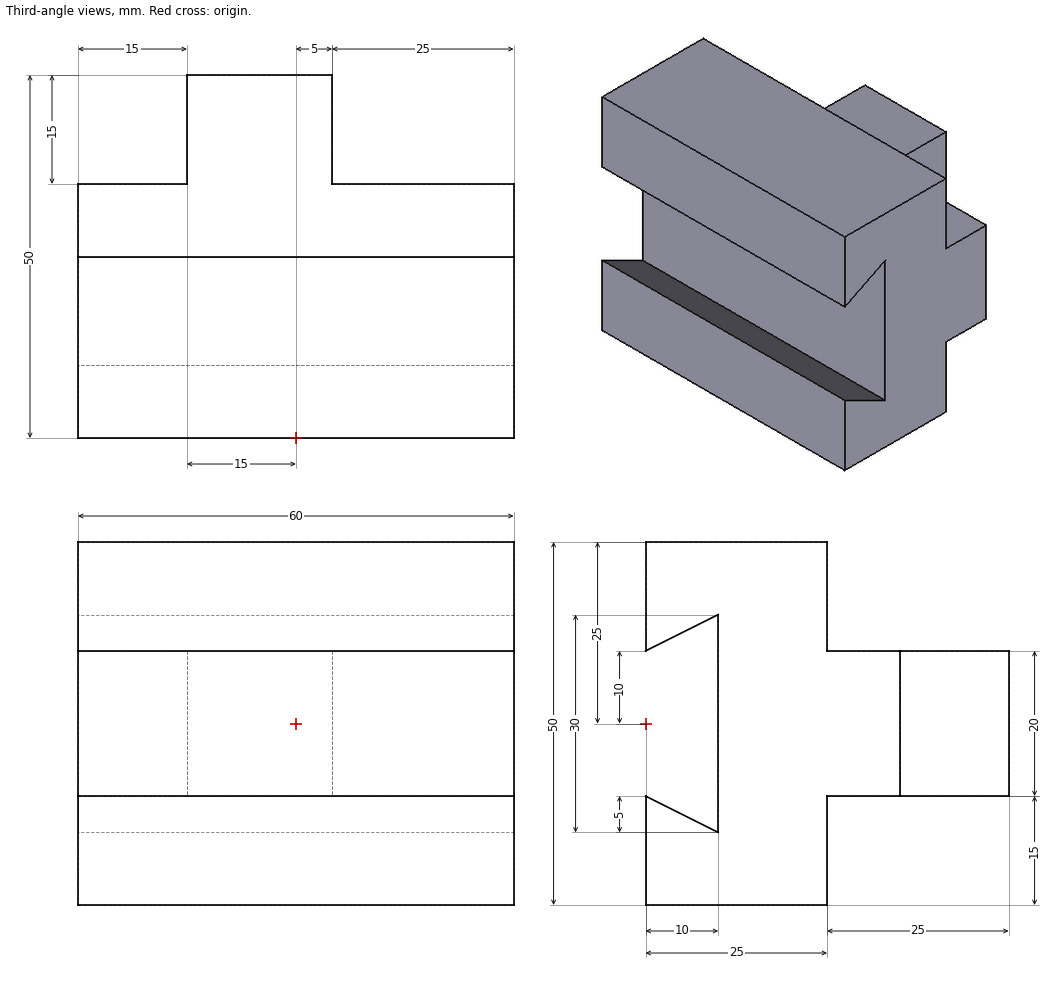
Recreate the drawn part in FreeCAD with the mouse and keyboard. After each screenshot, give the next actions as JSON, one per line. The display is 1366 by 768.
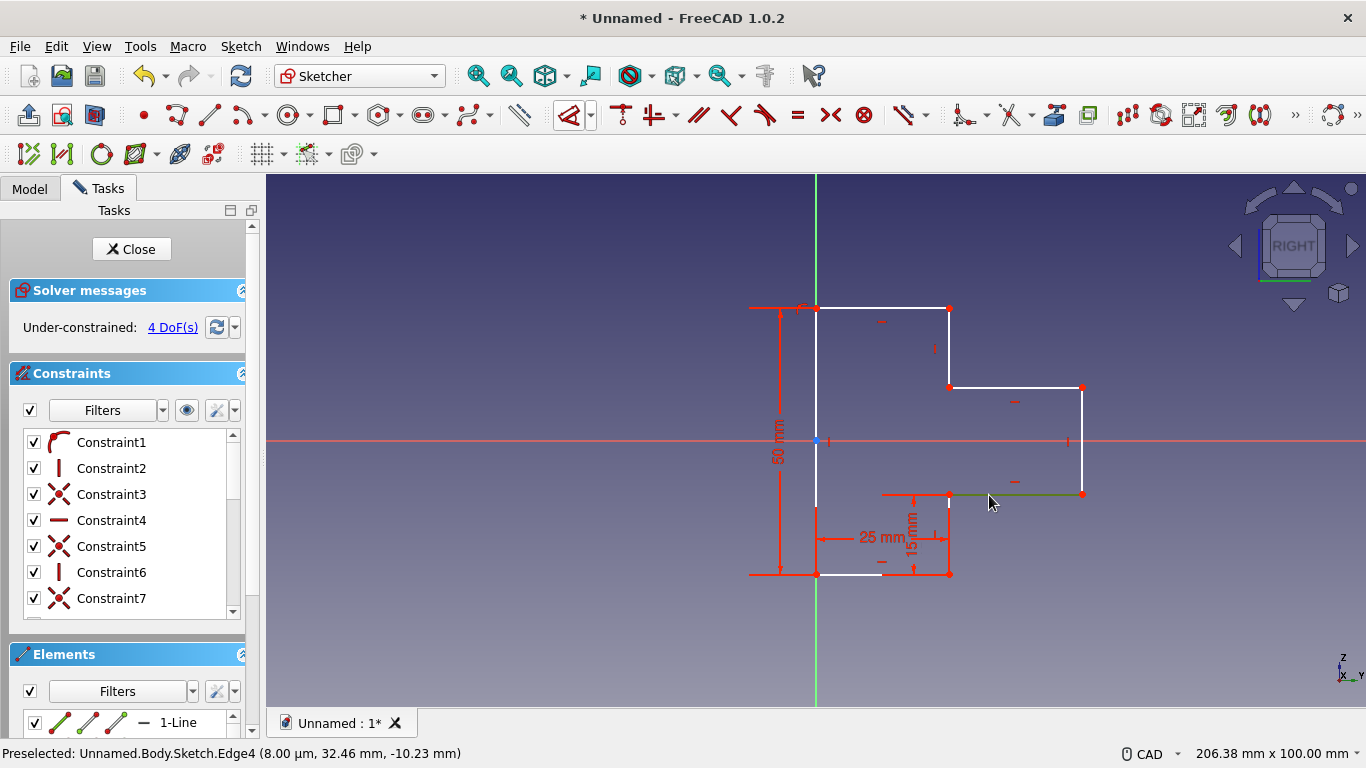
{"action": "key", "text": "l"}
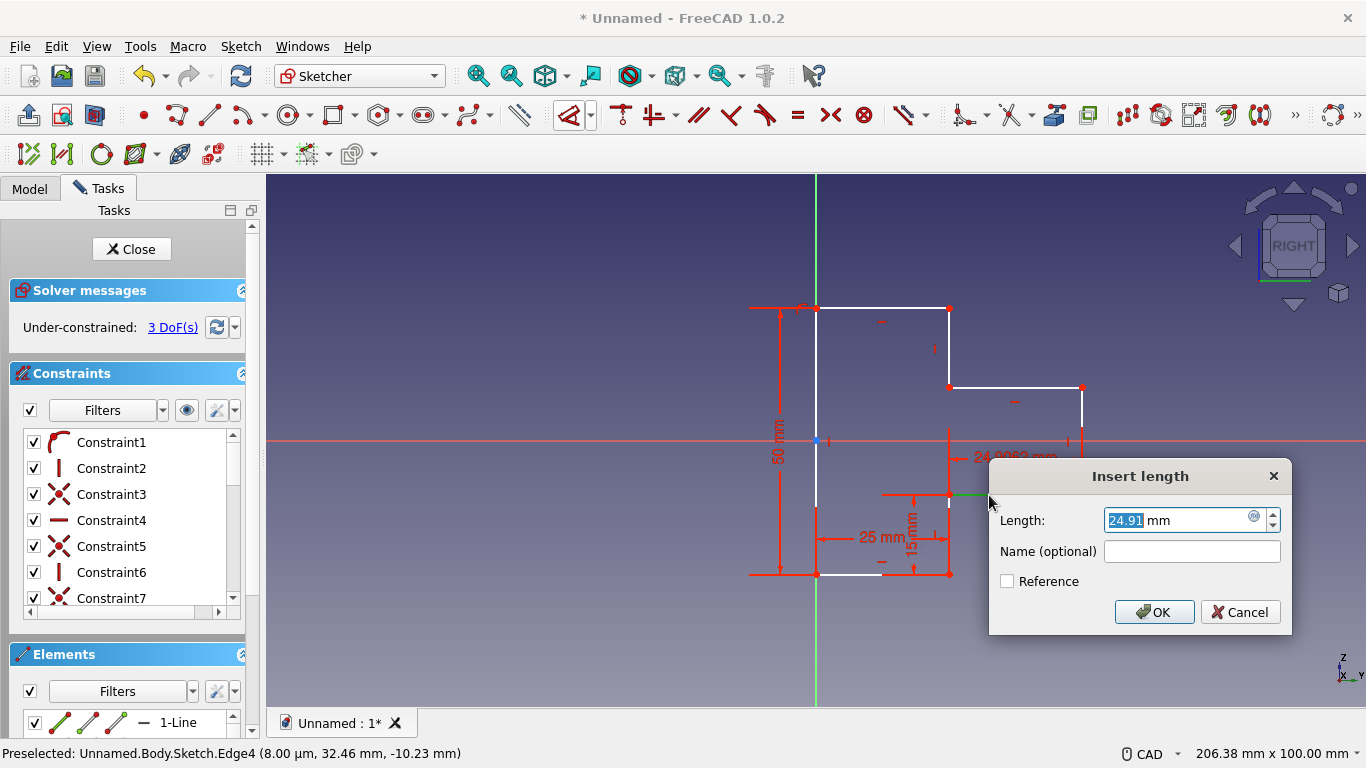
{"action": "type", "text": "25"}
{"action": "key", "text": "Return"}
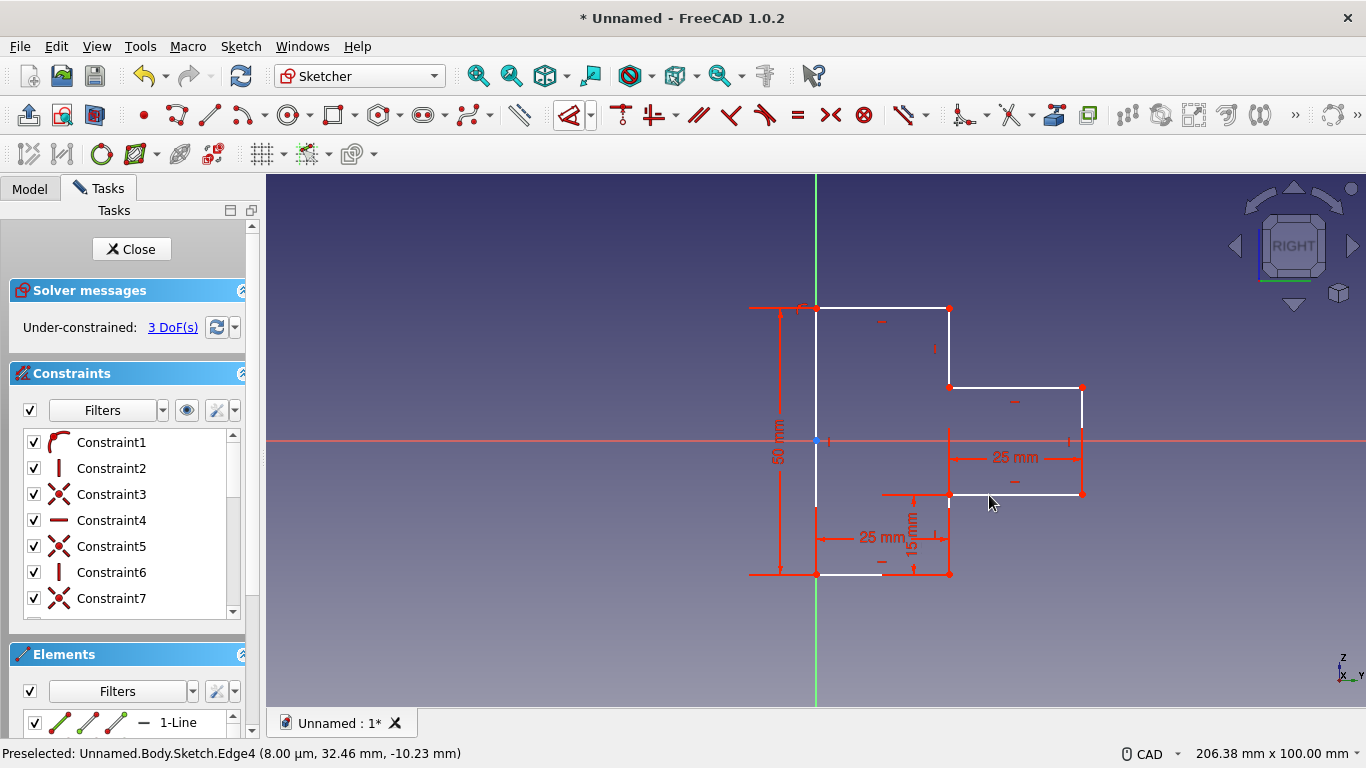
{"action": "left_click", "coordinate": [1082, 463]}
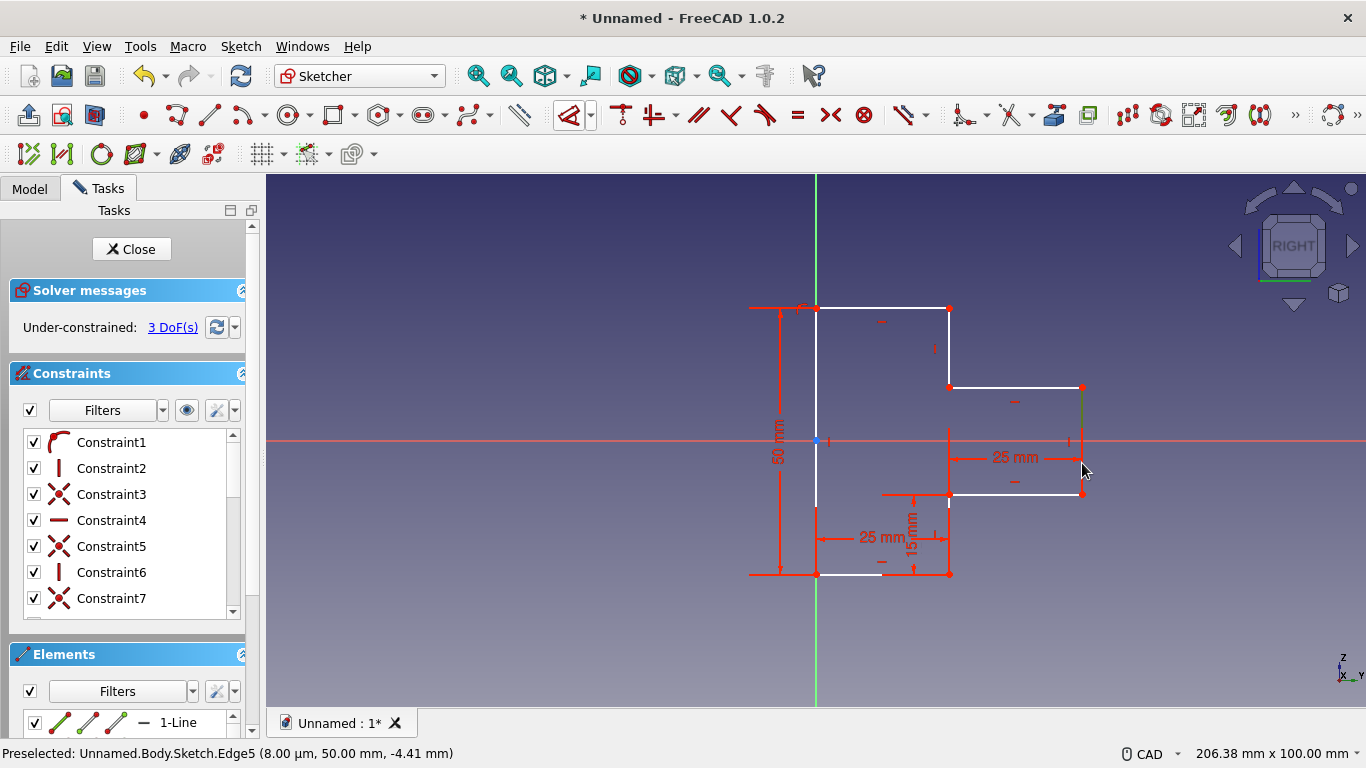
{"action": "left_click", "coordinate": [590, 116]}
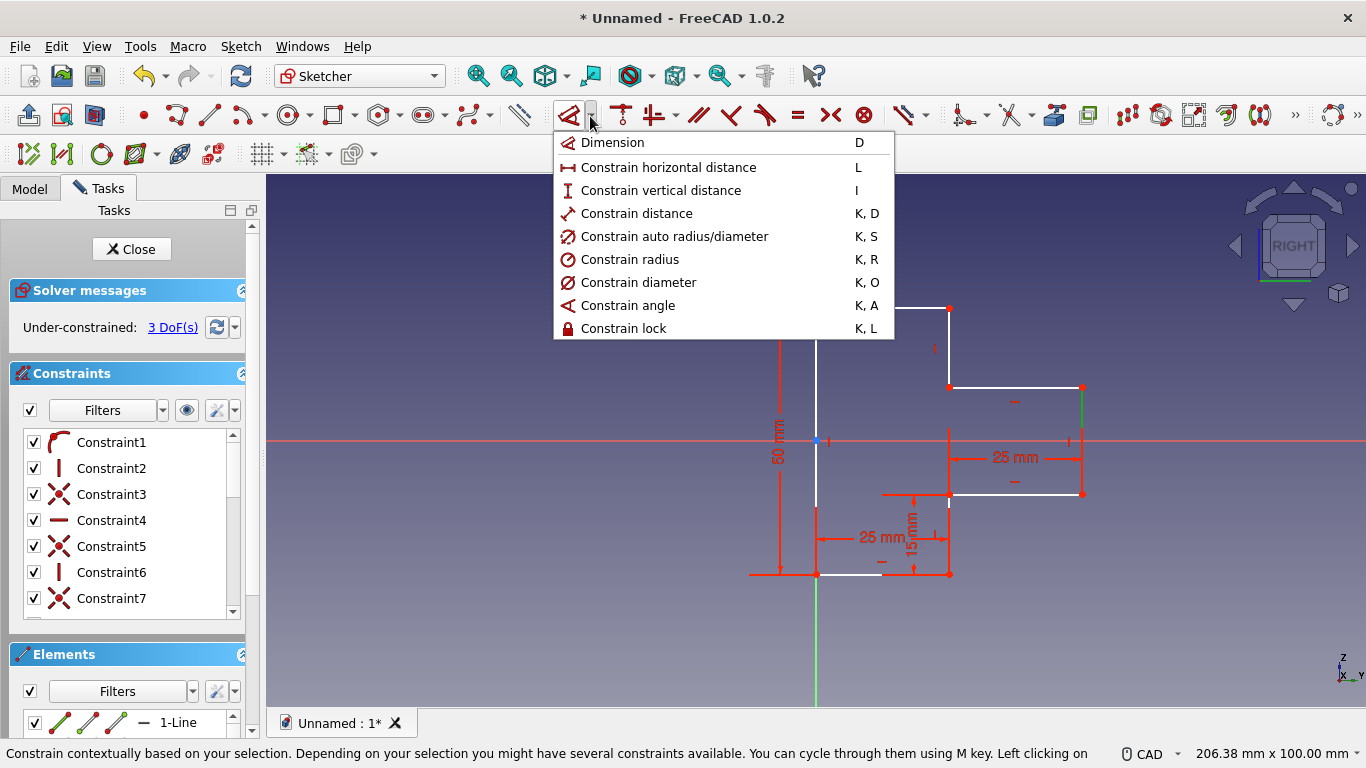
{"action": "left_click", "coordinate": [724, 190]}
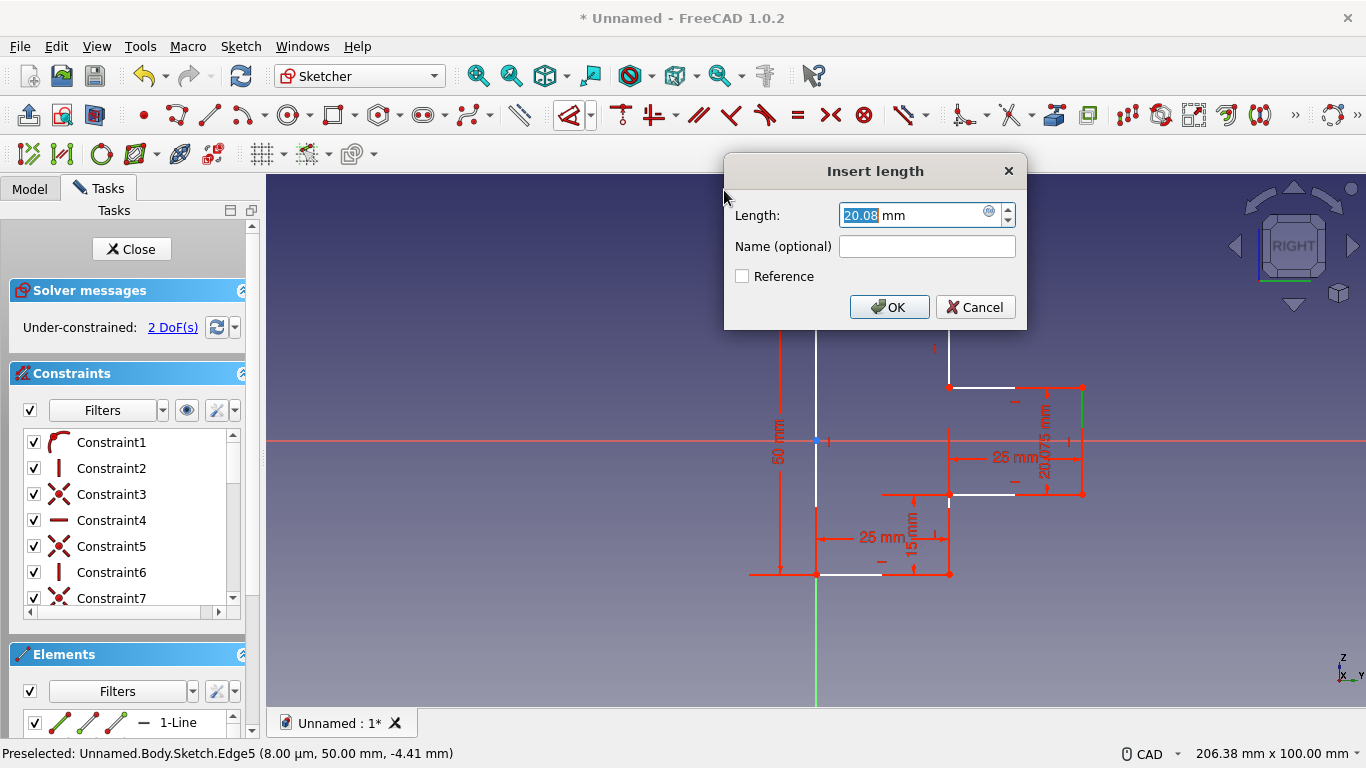
{"action": "type", "text": "20"}
{"action": "key", "text": "Return"}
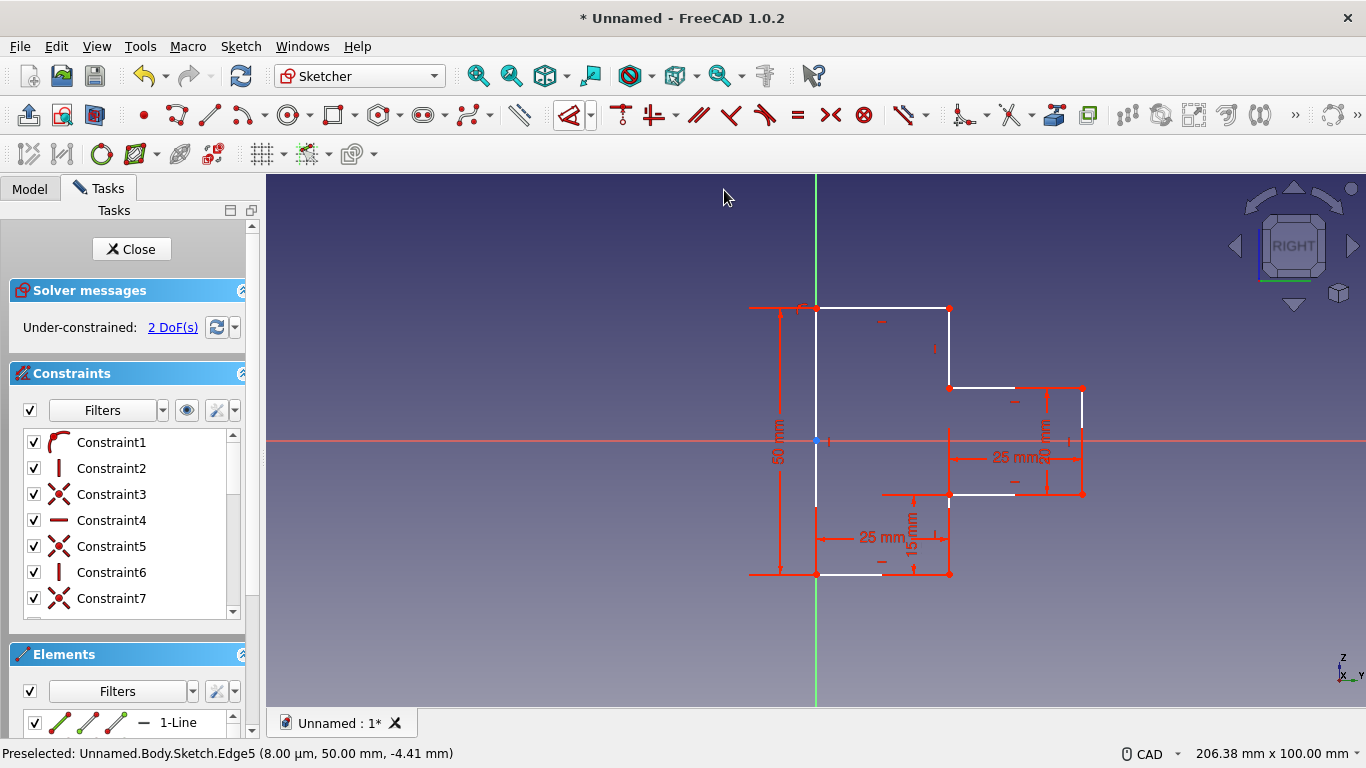
{"action": "left_click", "coordinate": [1042, 388]}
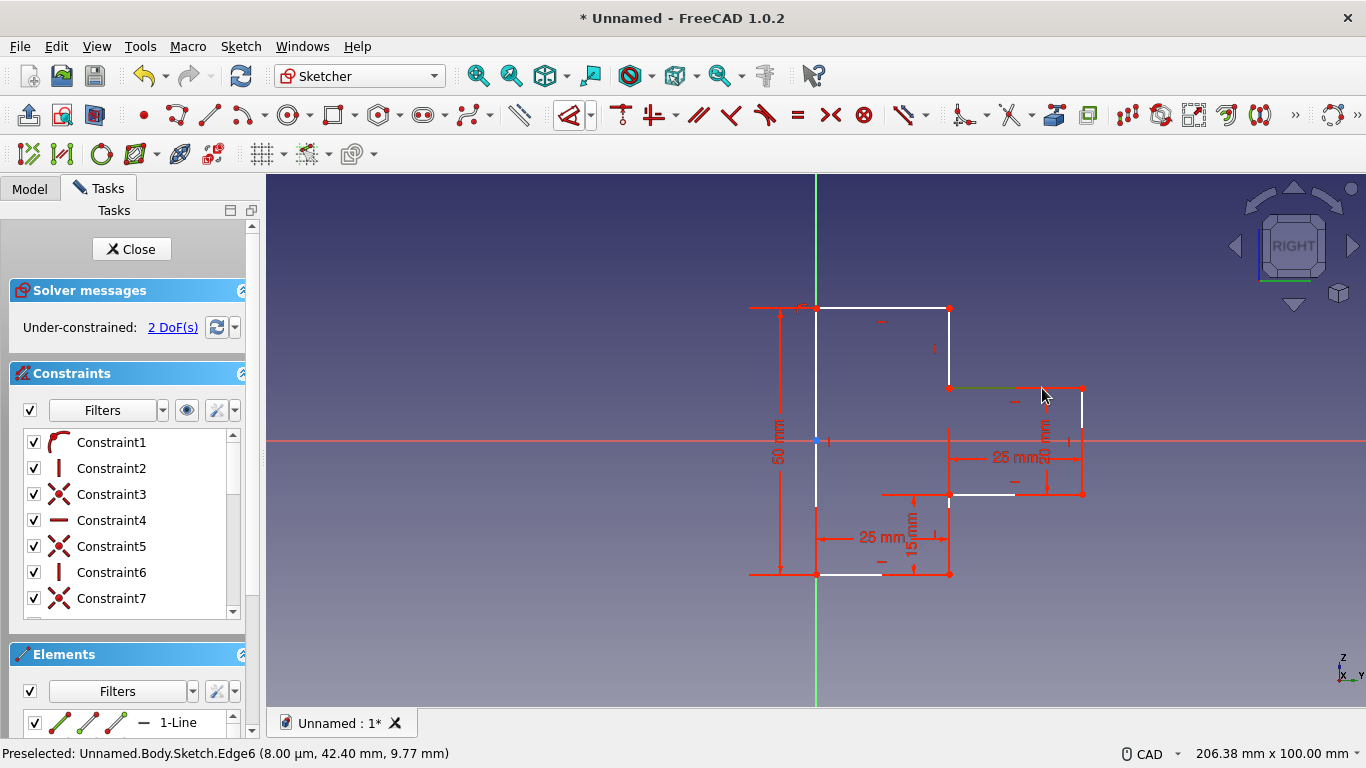
{"action": "key", "text": "l"}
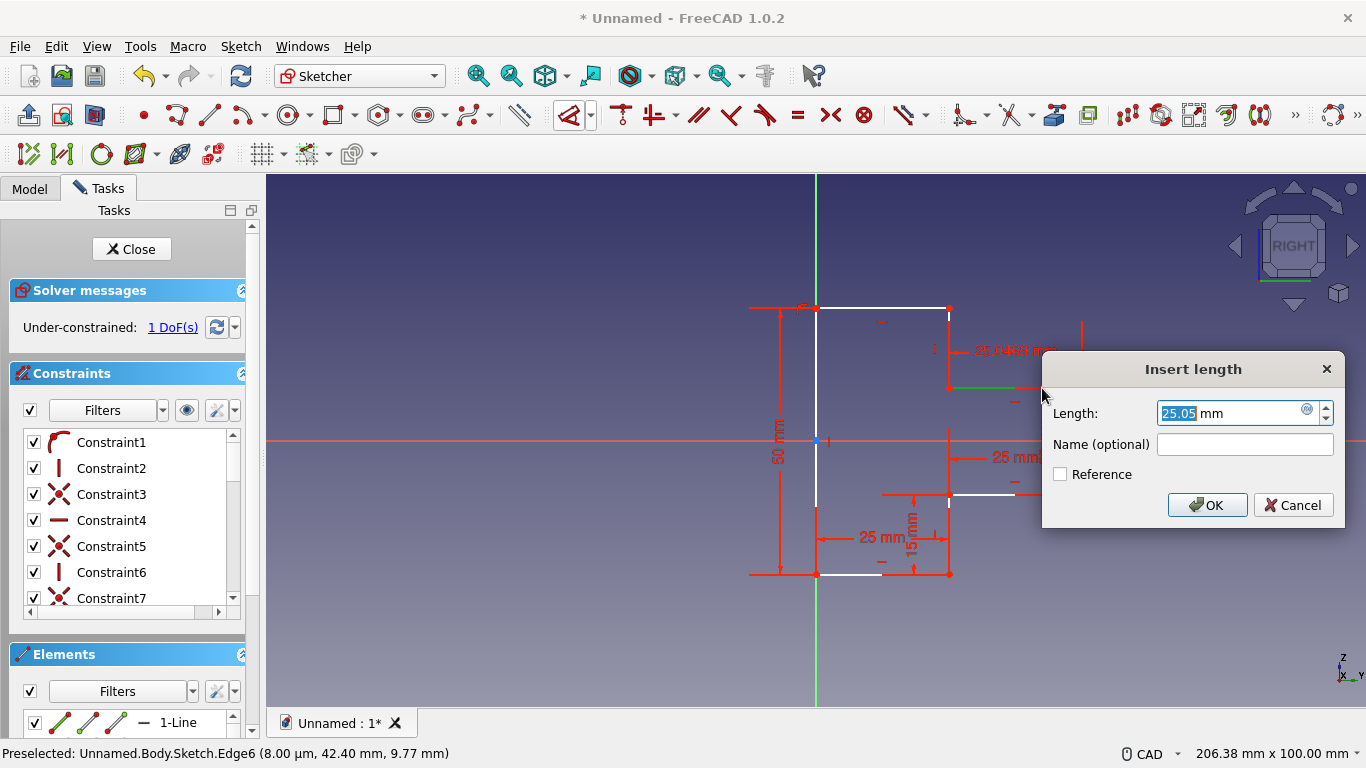
{"action": "type", "text": "25"}
{"action": "key", "text": "Return"}